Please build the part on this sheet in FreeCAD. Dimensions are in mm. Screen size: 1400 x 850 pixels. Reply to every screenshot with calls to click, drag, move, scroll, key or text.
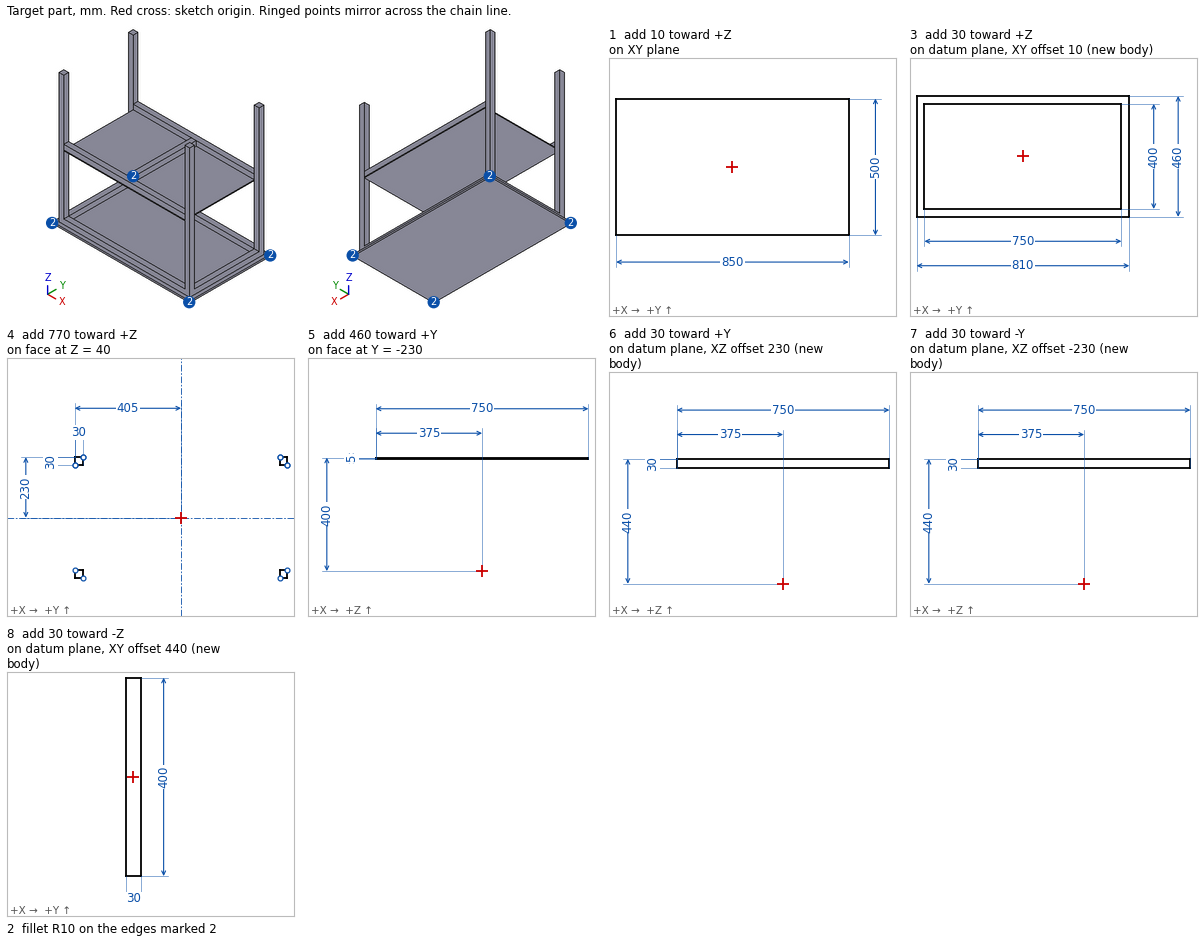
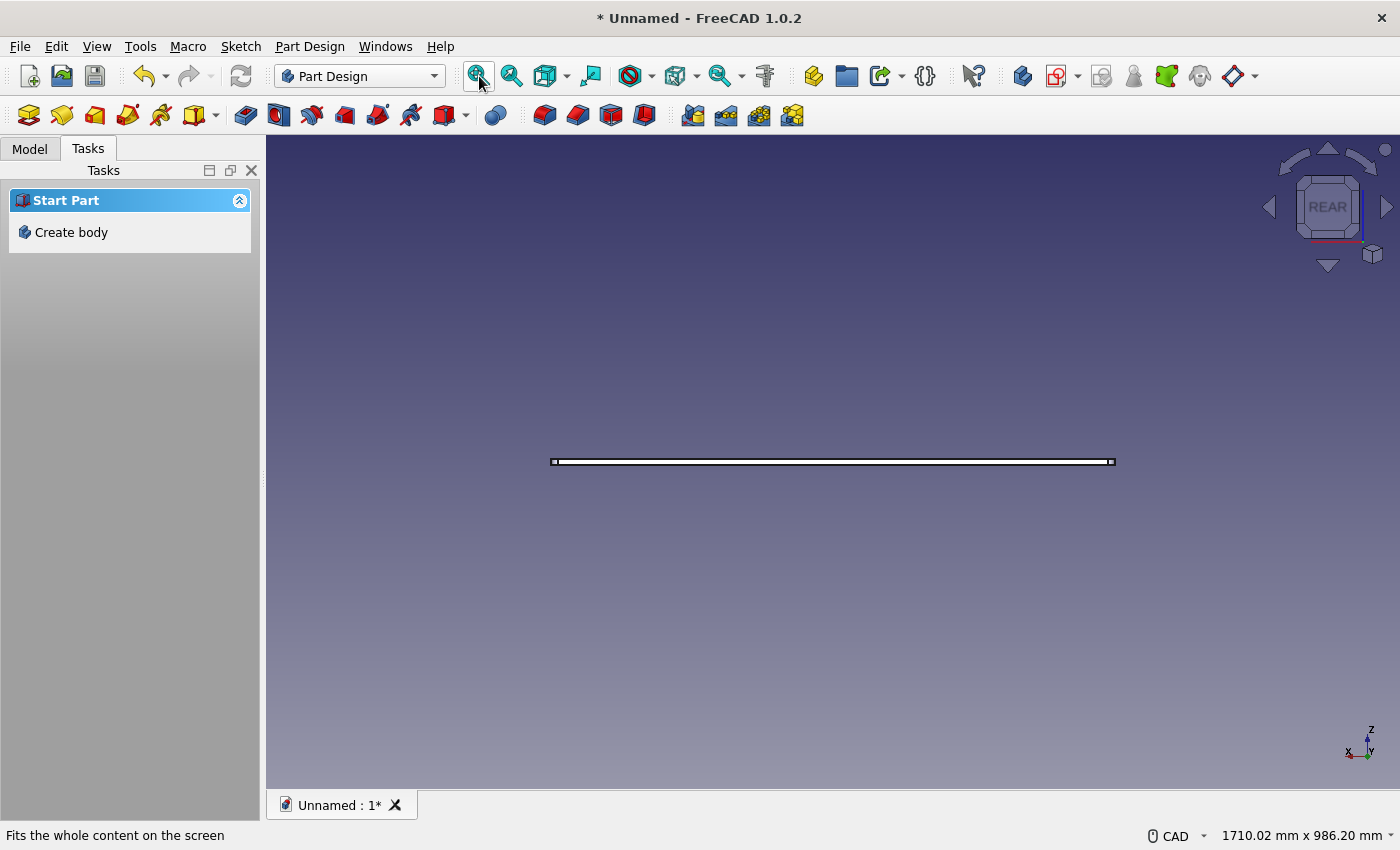
click(1023, 76)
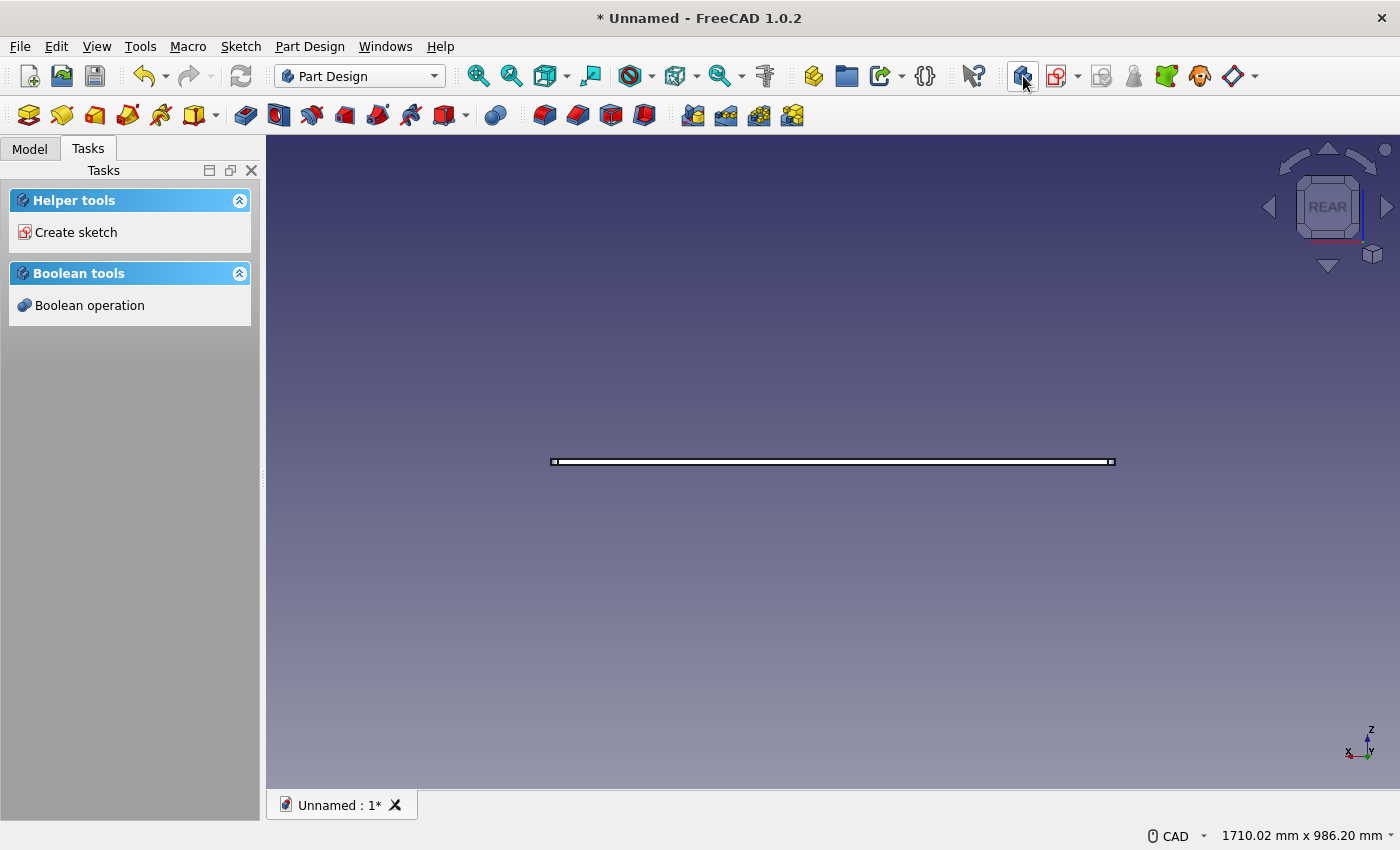
click(30, 148)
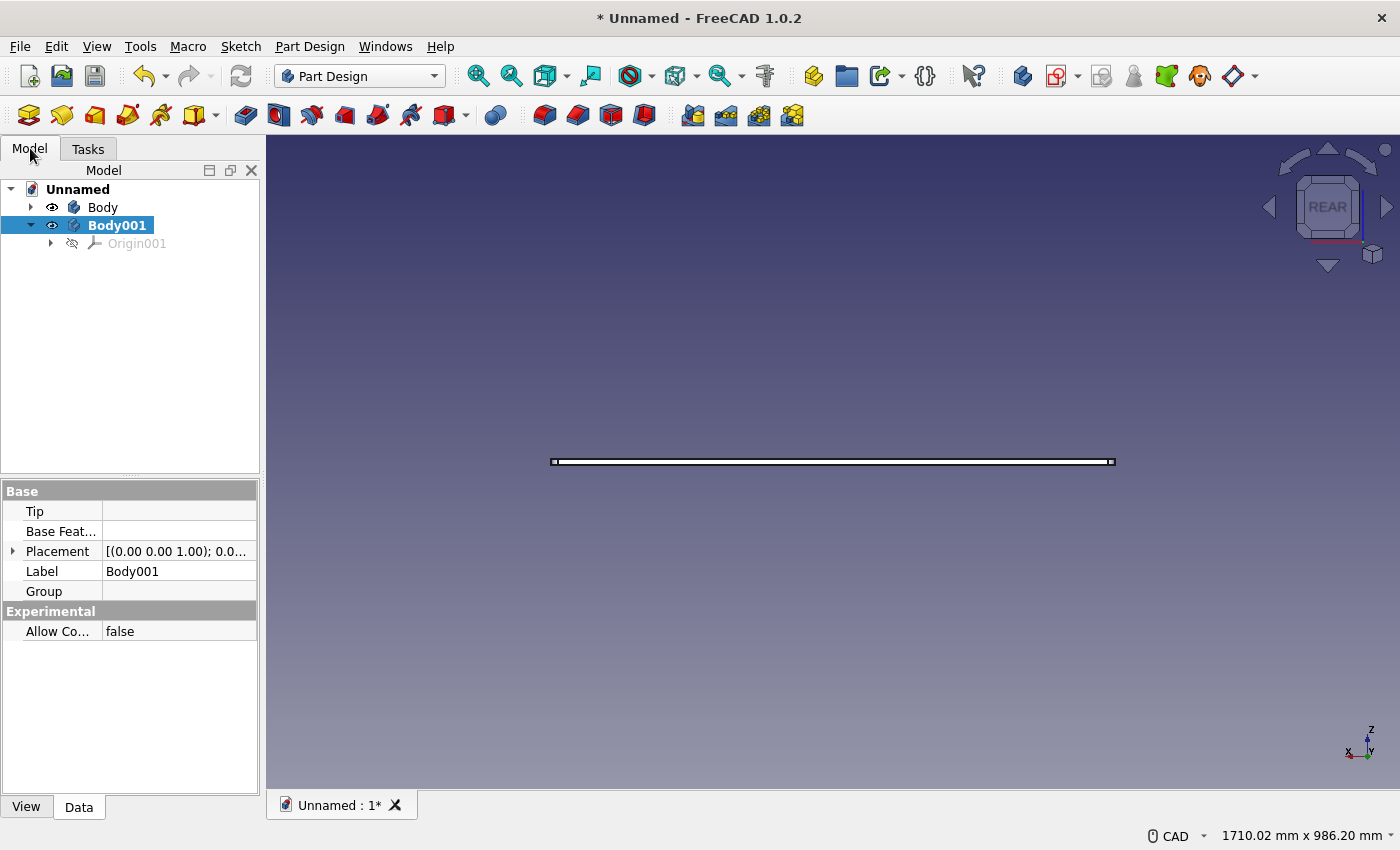
click(51, 243)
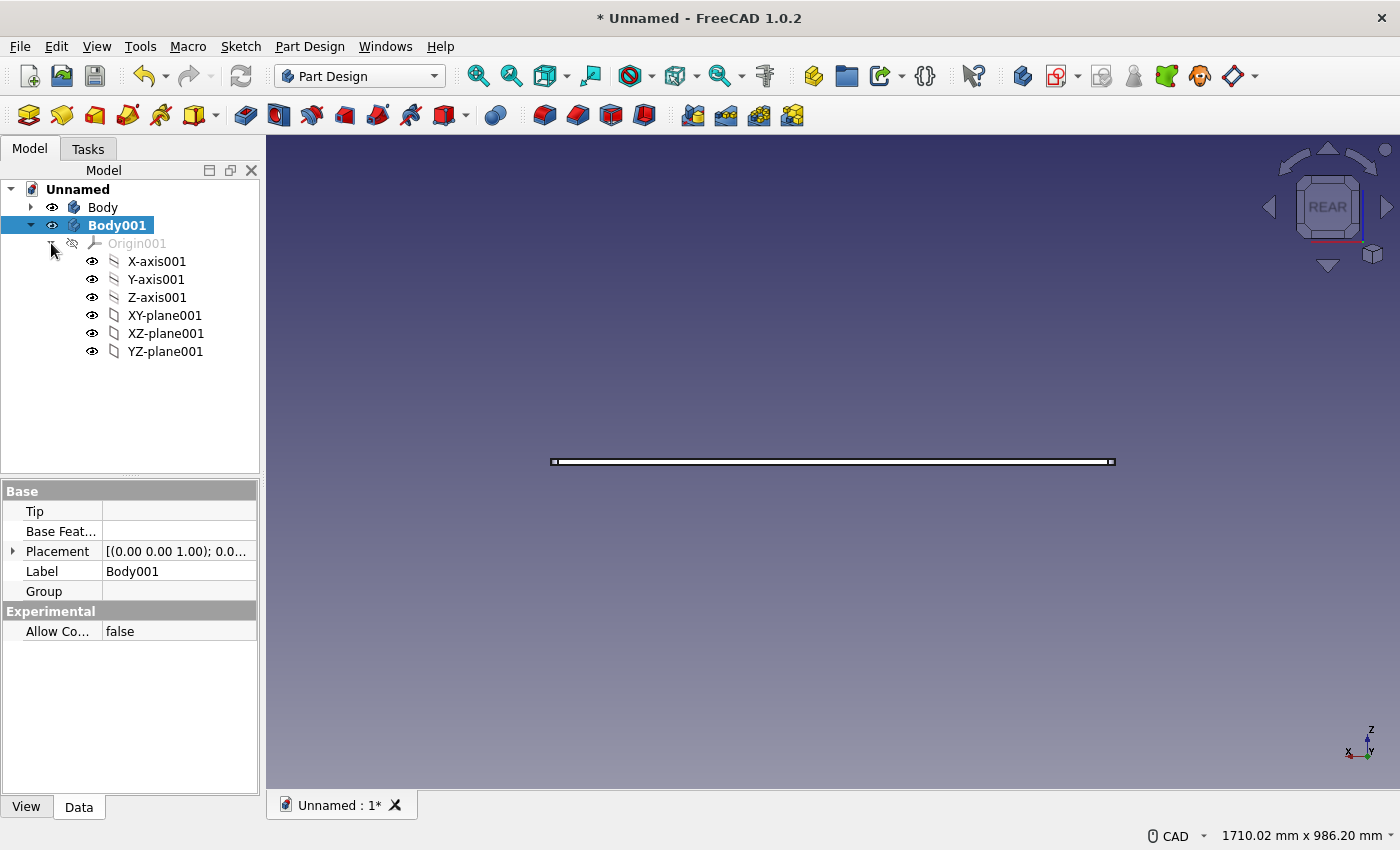
click(137, 315)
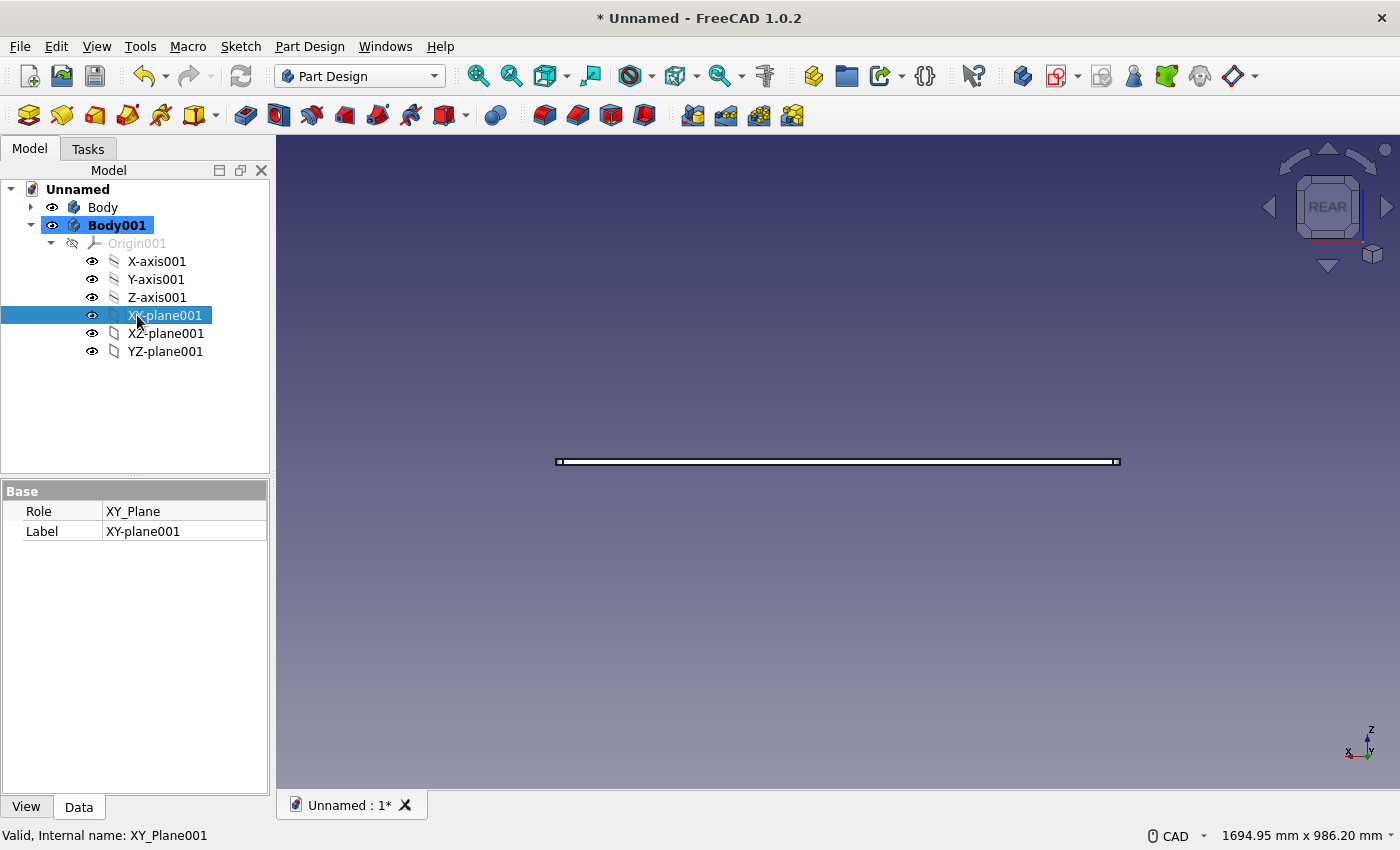
click(1232, 76)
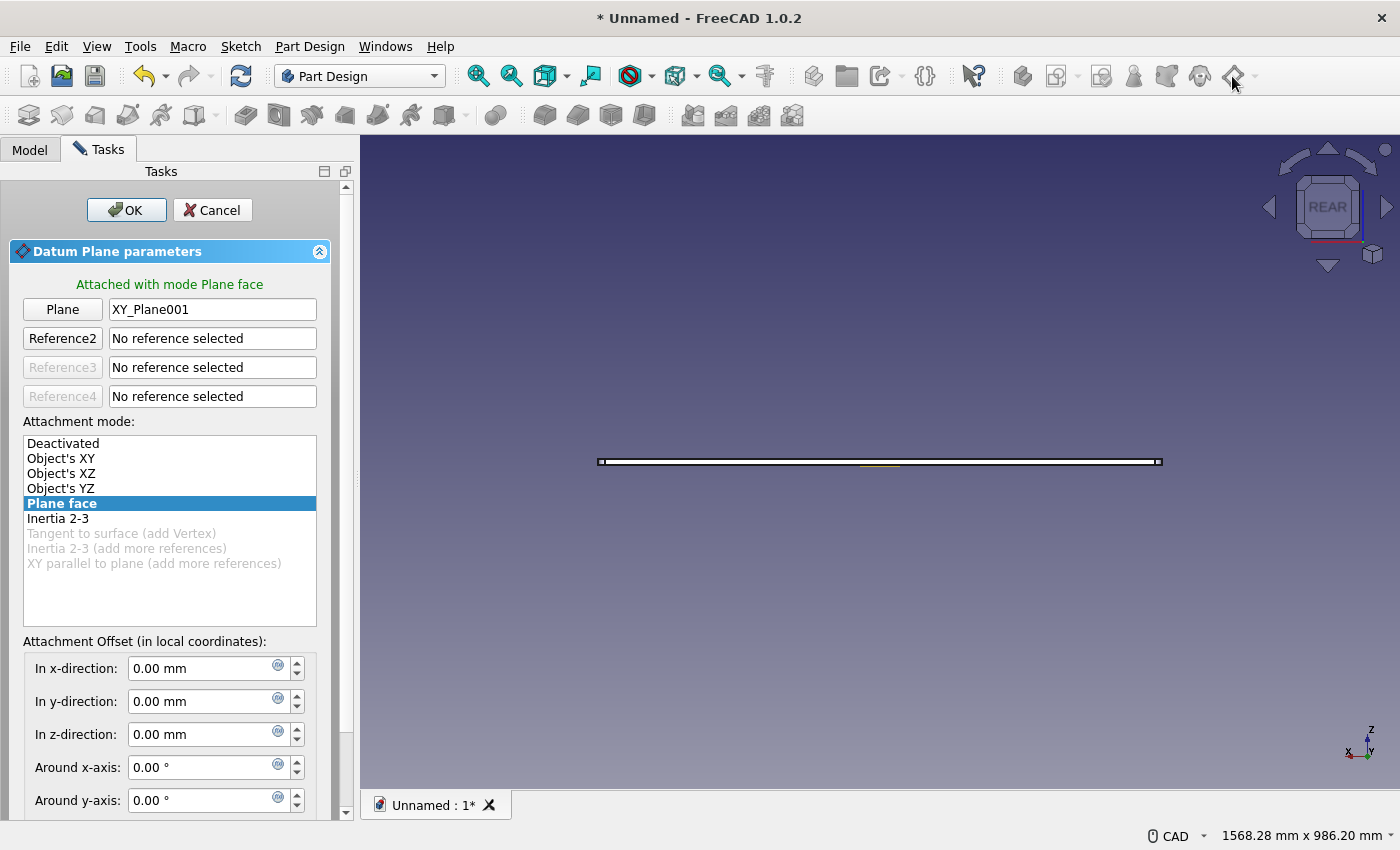
triple_click(210, 734)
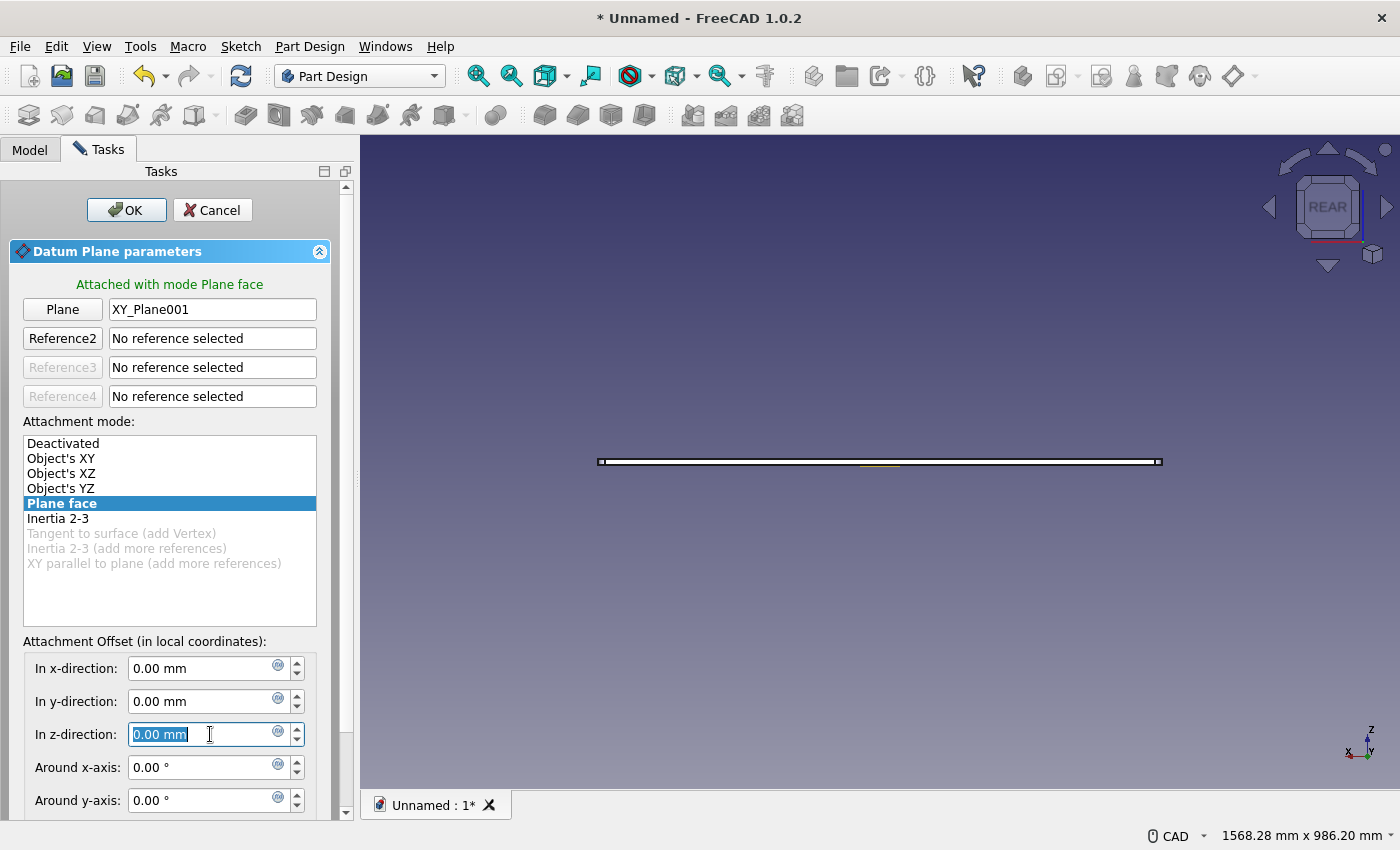
text(10)
key(Tab)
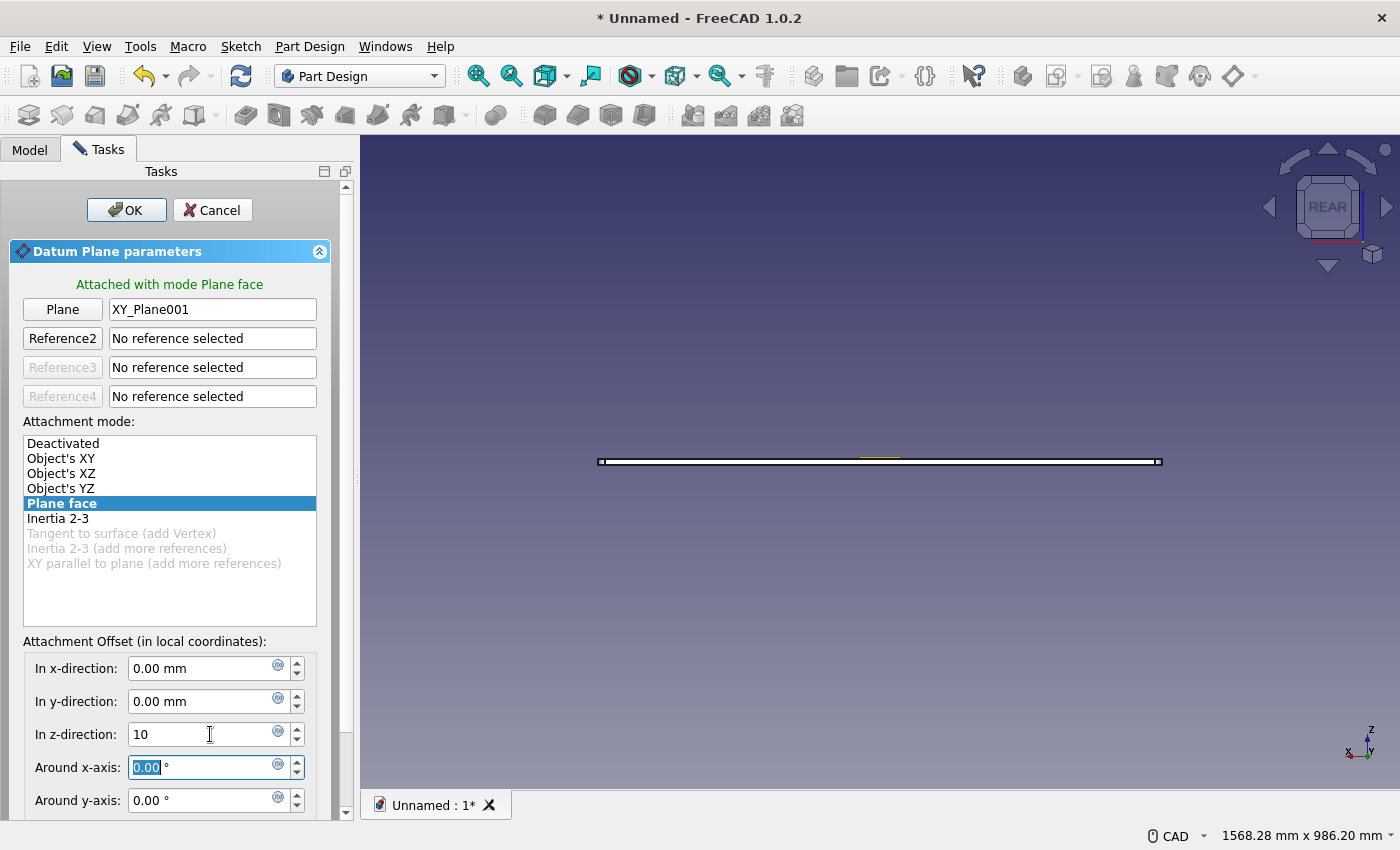
click(127, 210)